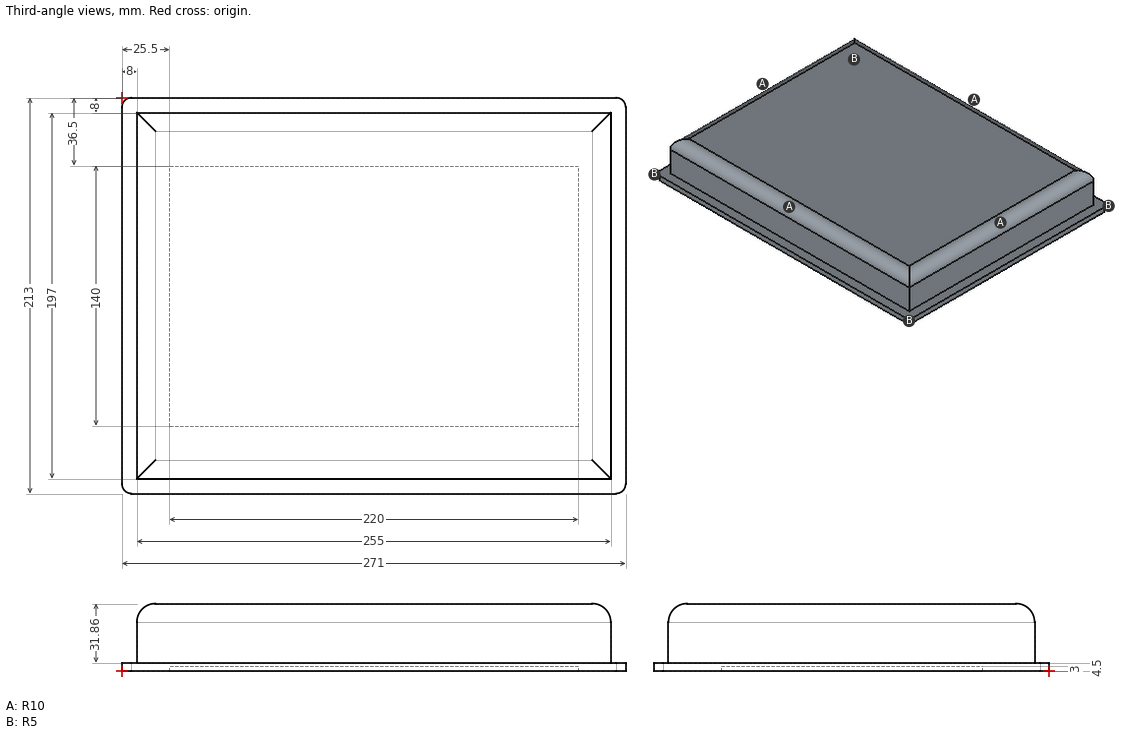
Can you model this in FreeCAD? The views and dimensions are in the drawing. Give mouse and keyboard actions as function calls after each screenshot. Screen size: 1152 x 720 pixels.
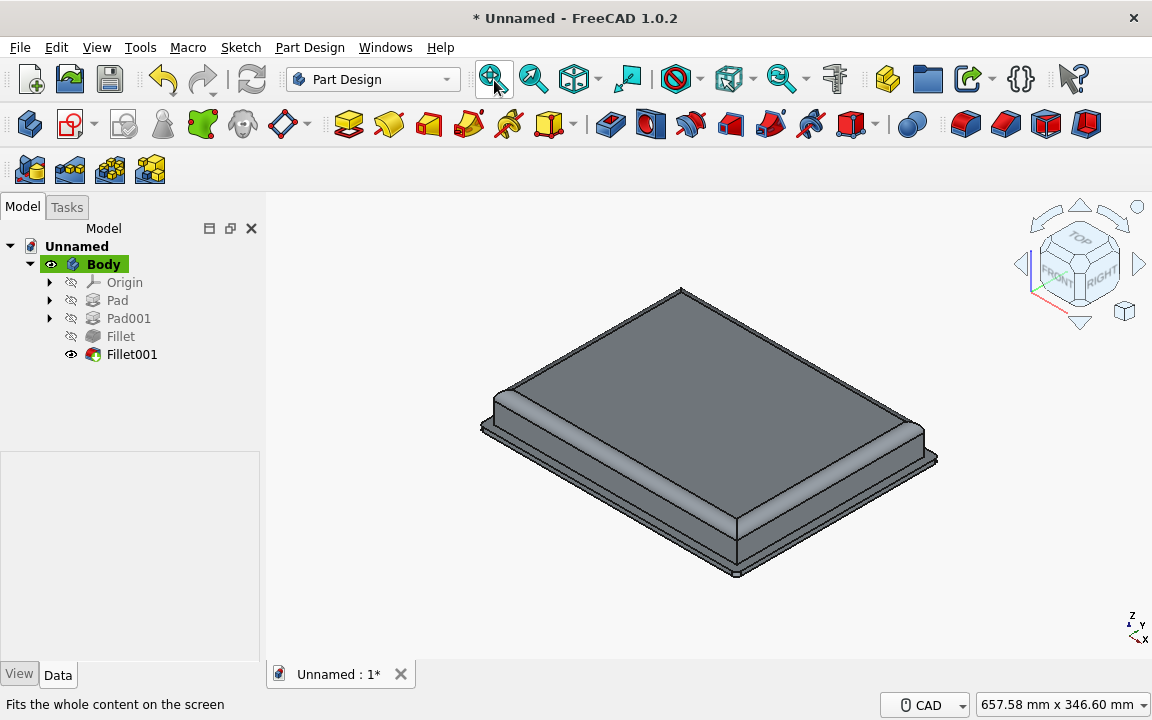
click(70, 124)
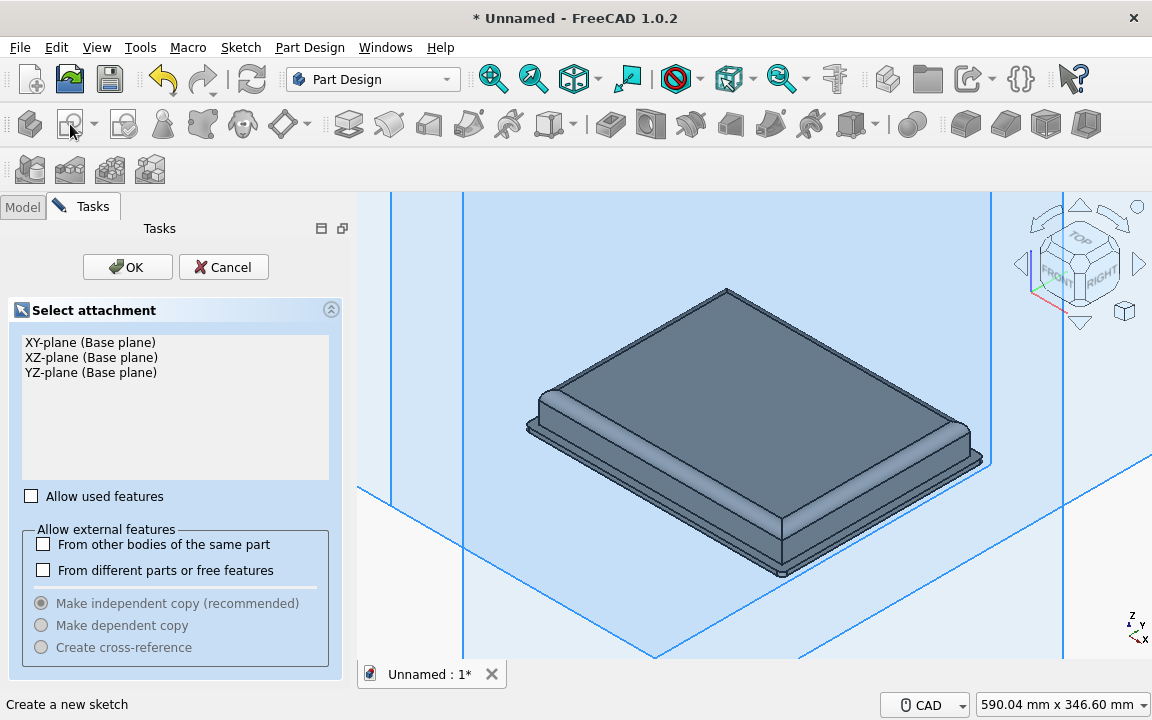
click(82, 342)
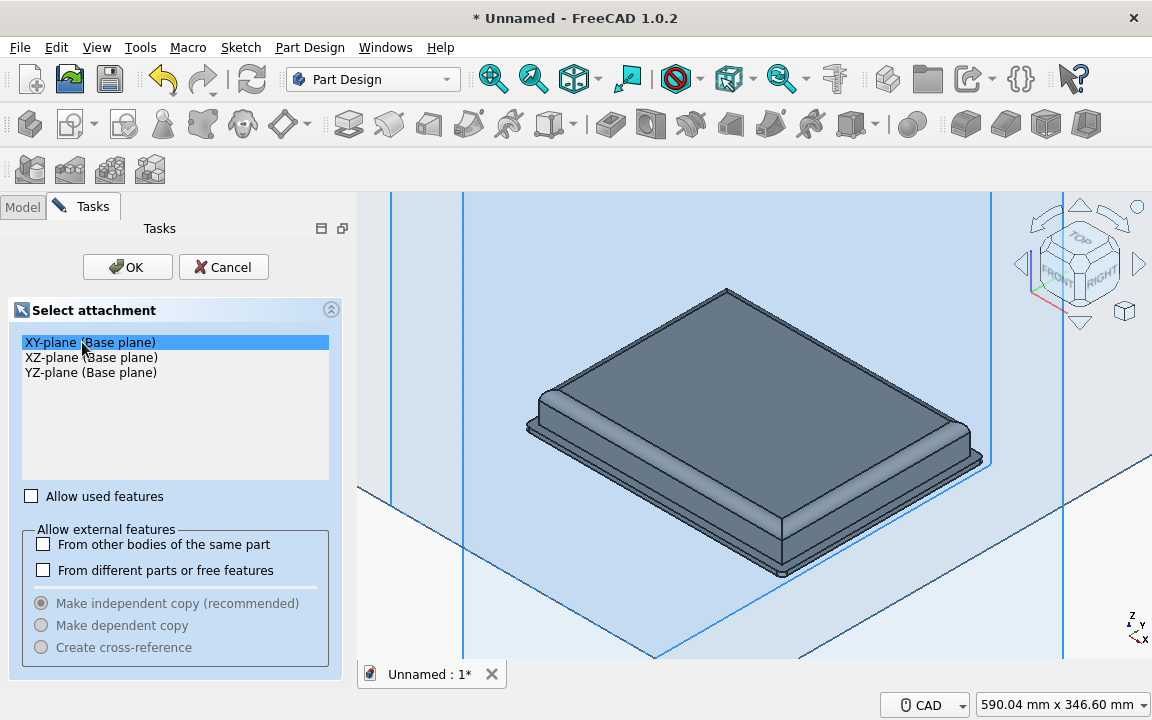
click(128, 267)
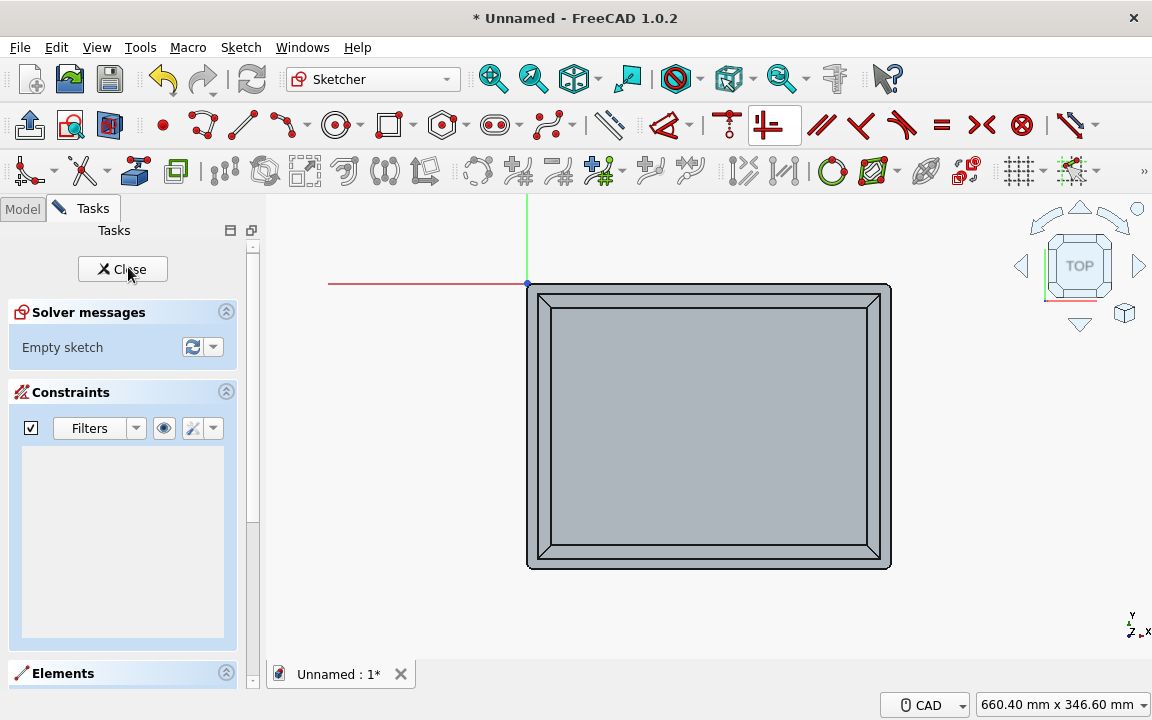
click(110, 126)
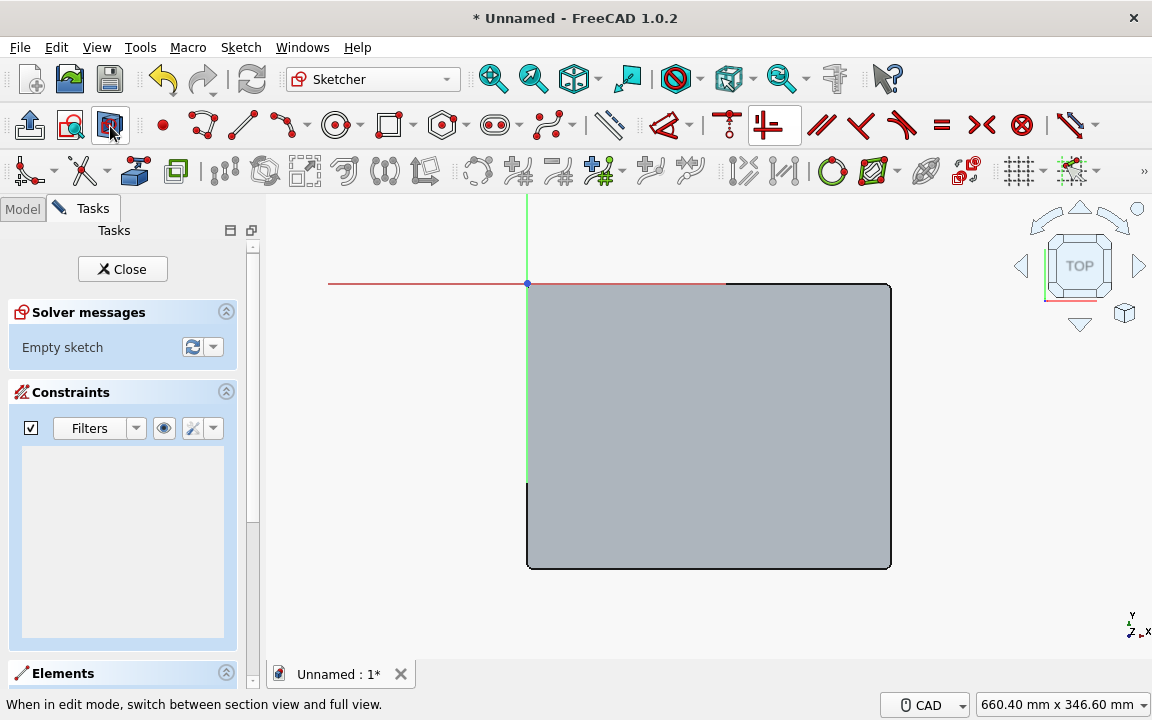
click(390, 126)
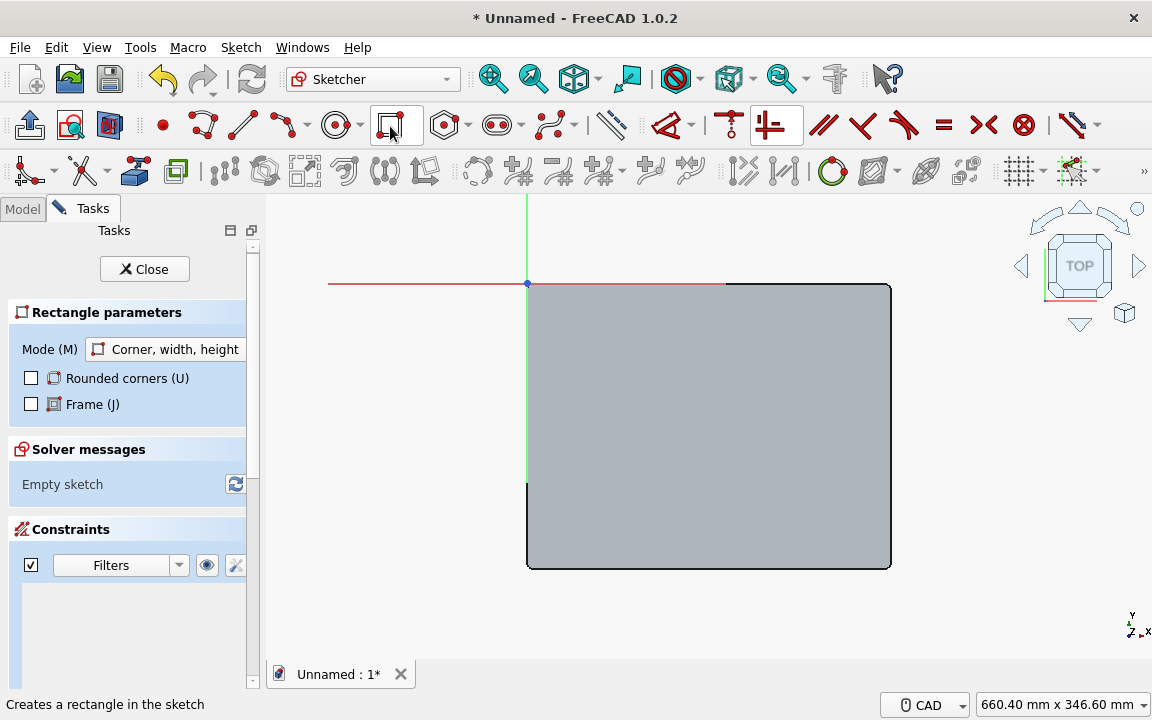
click(561, 333)
click(857, 520)
key(Escape)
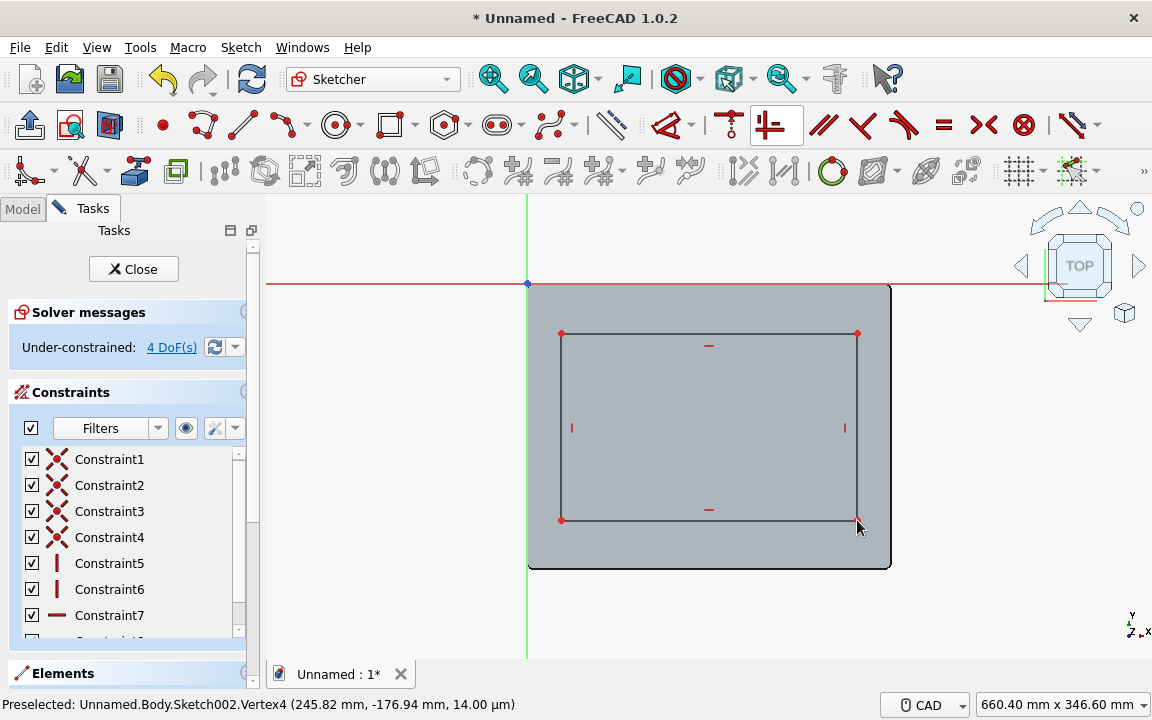
click(666, 126)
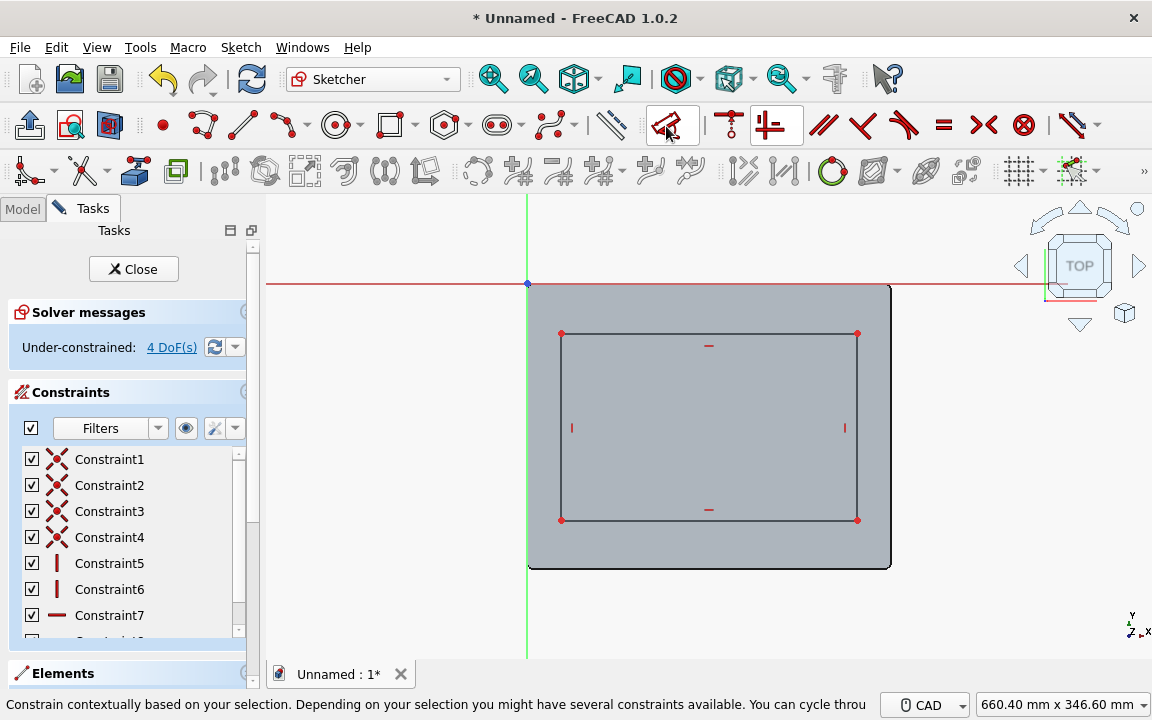
click(561, 390)
click(595, 428)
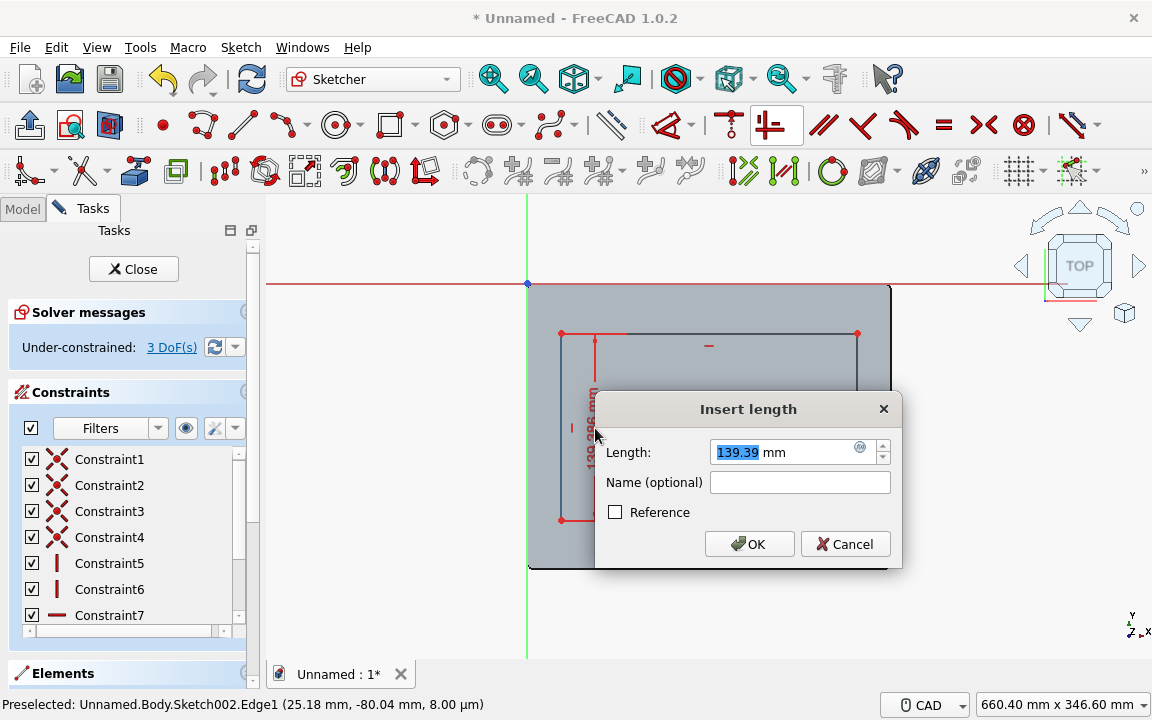
text(140)
key(Return)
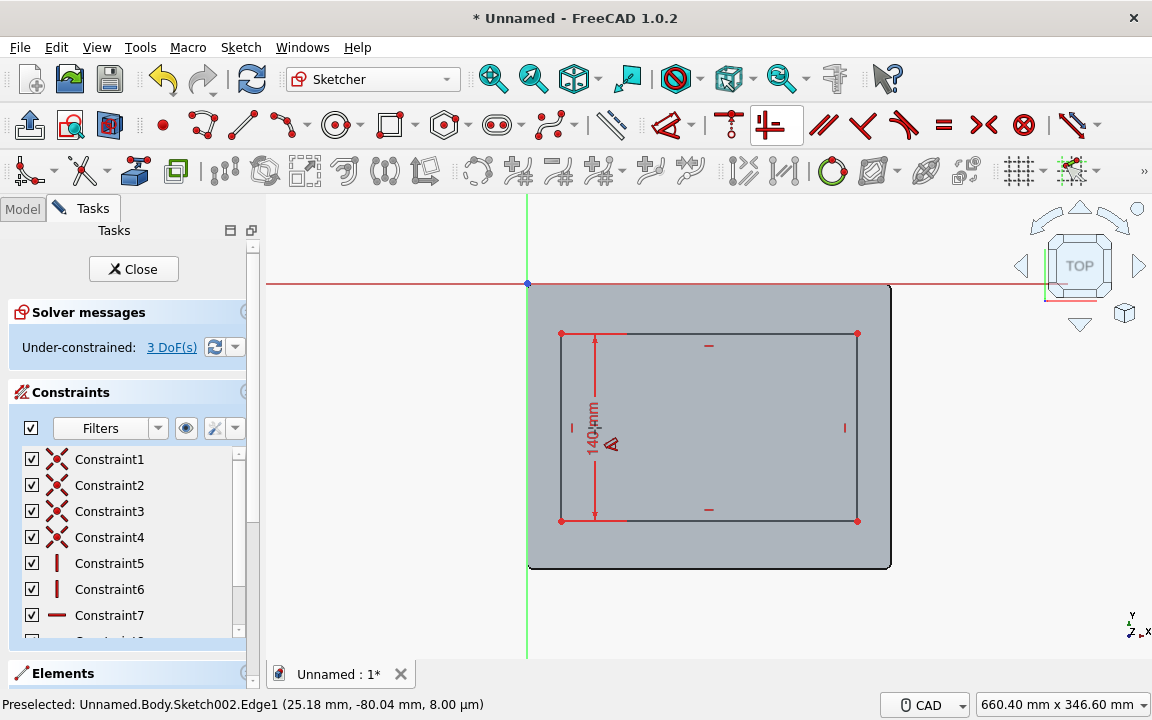
click(650, 521)
click(709, 555)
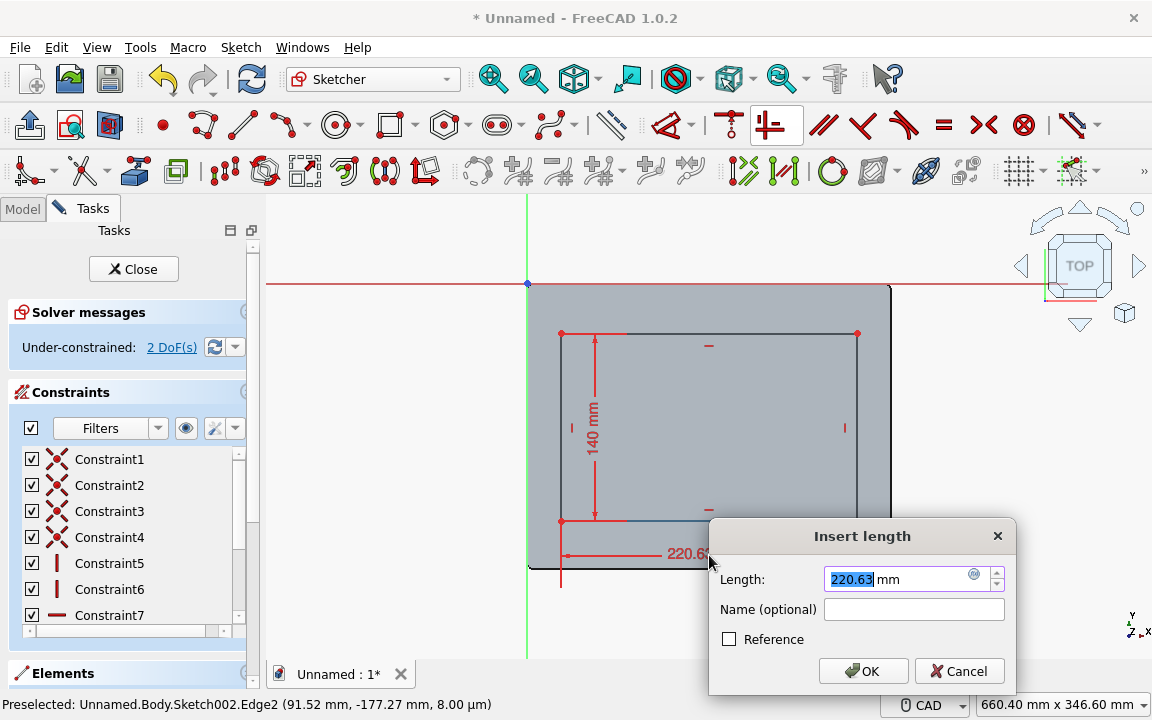
text(220)
key(Return)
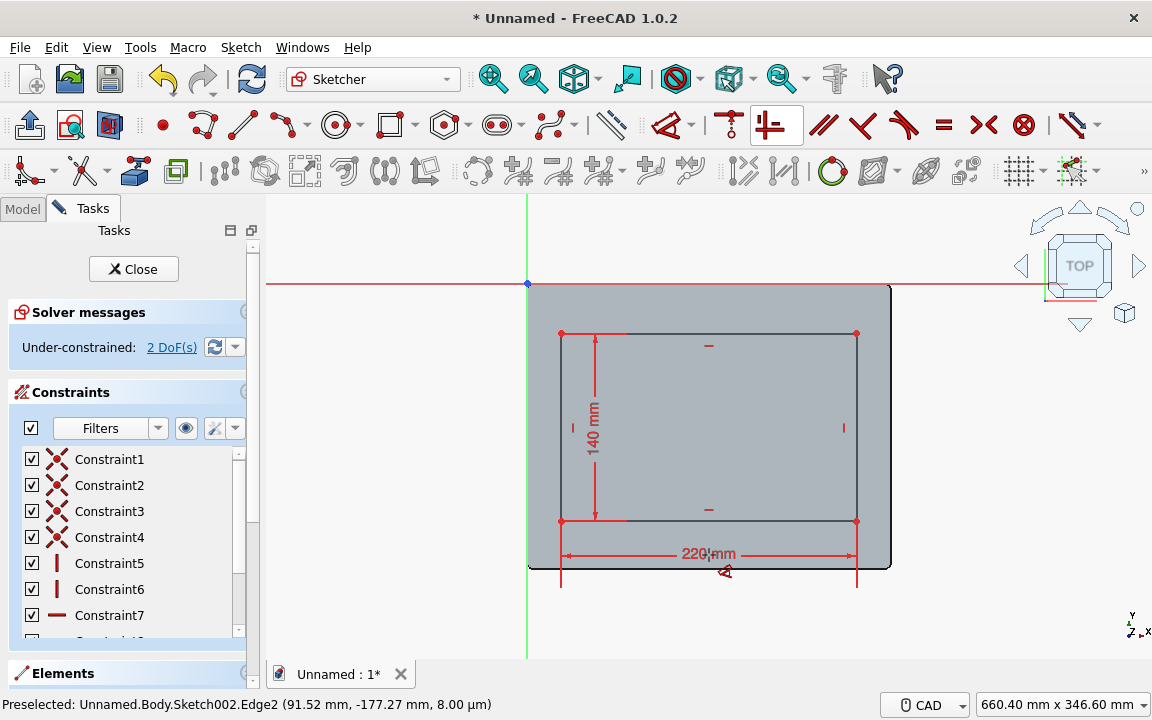
click(561, 334)
click(544, 250)